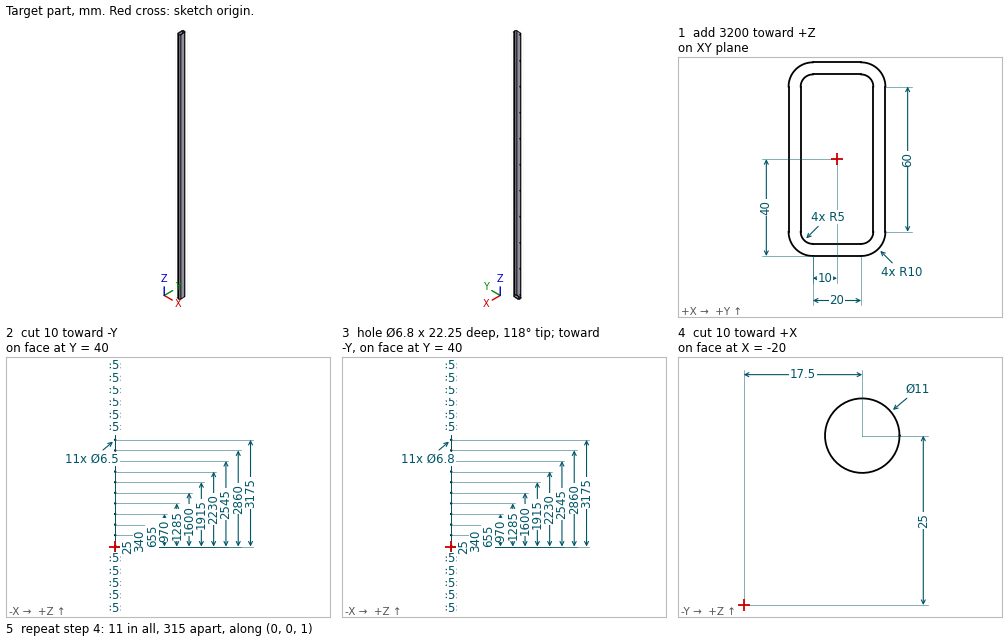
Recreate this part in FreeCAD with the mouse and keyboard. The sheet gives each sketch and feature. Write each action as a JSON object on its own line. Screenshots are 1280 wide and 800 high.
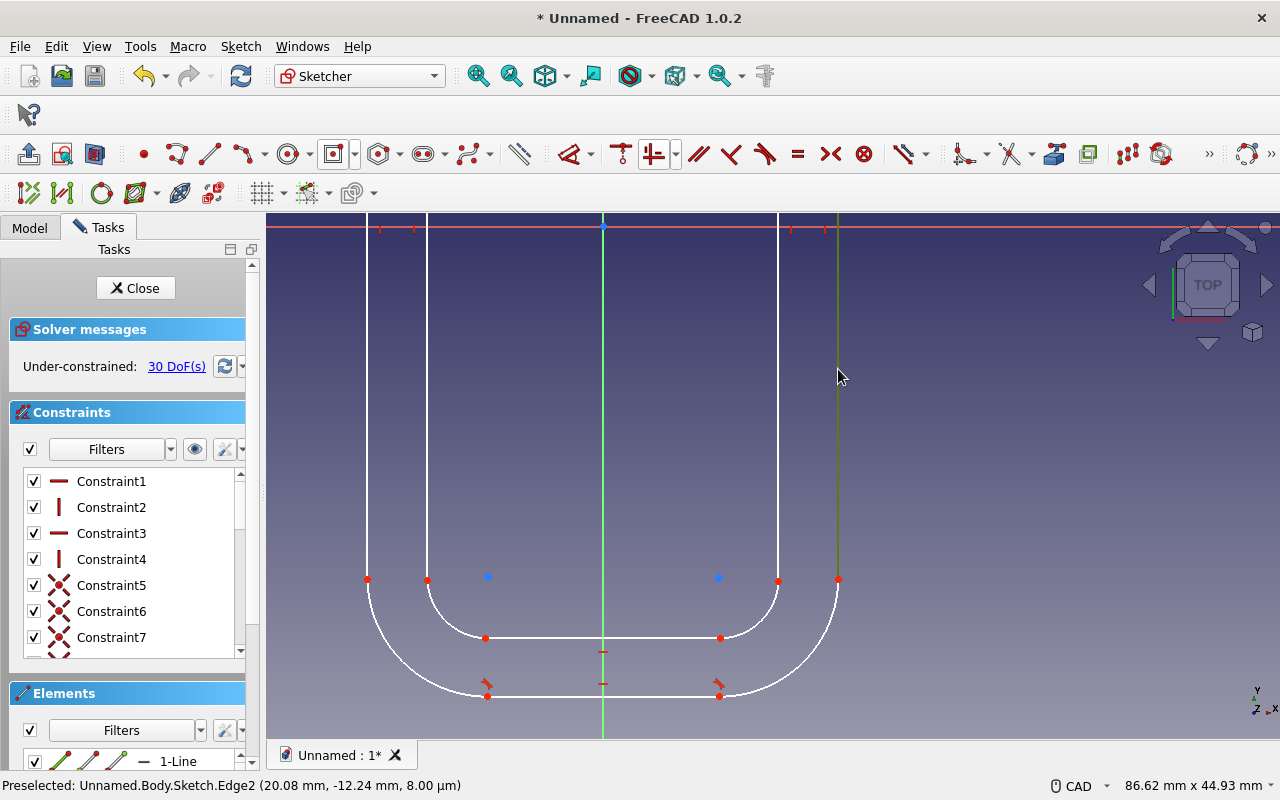
{"action": "left_click", "coordinate": [773, 684]}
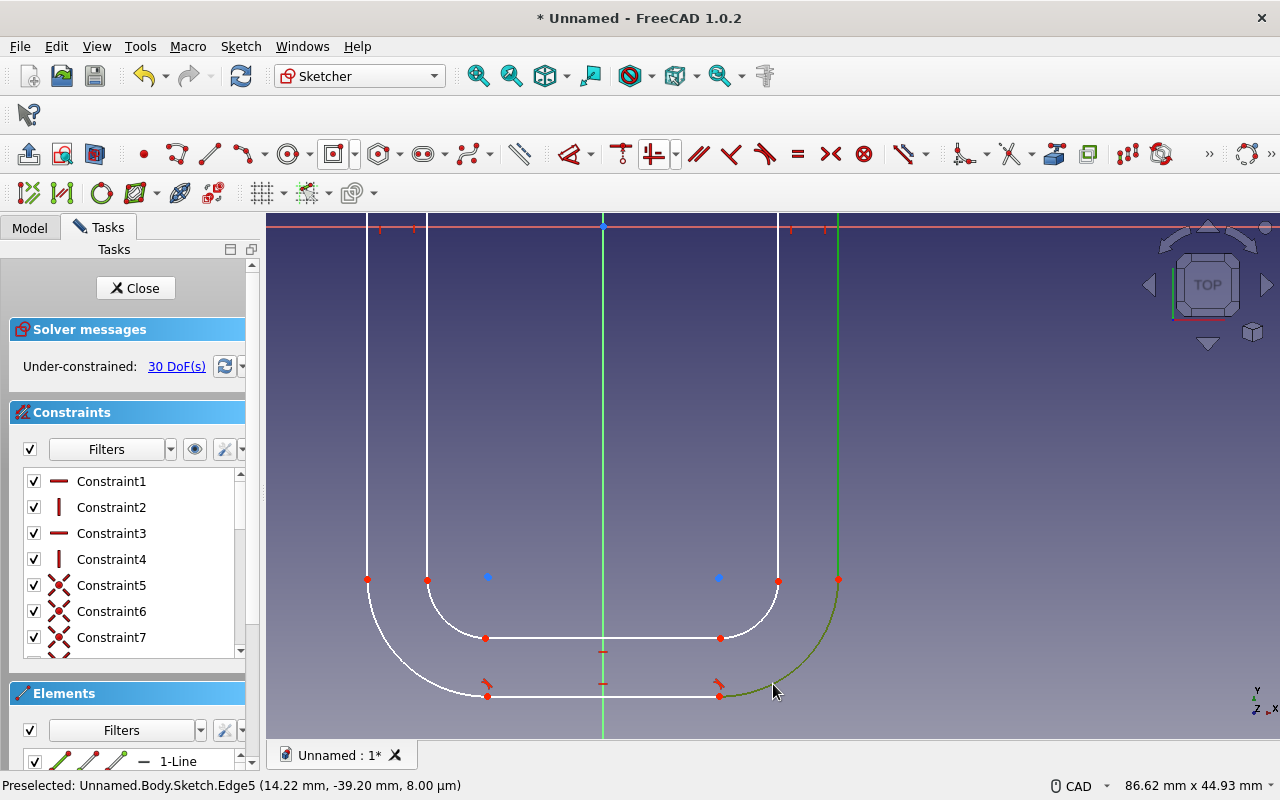
{"action": "left_click", "coordinate": [765, 154]}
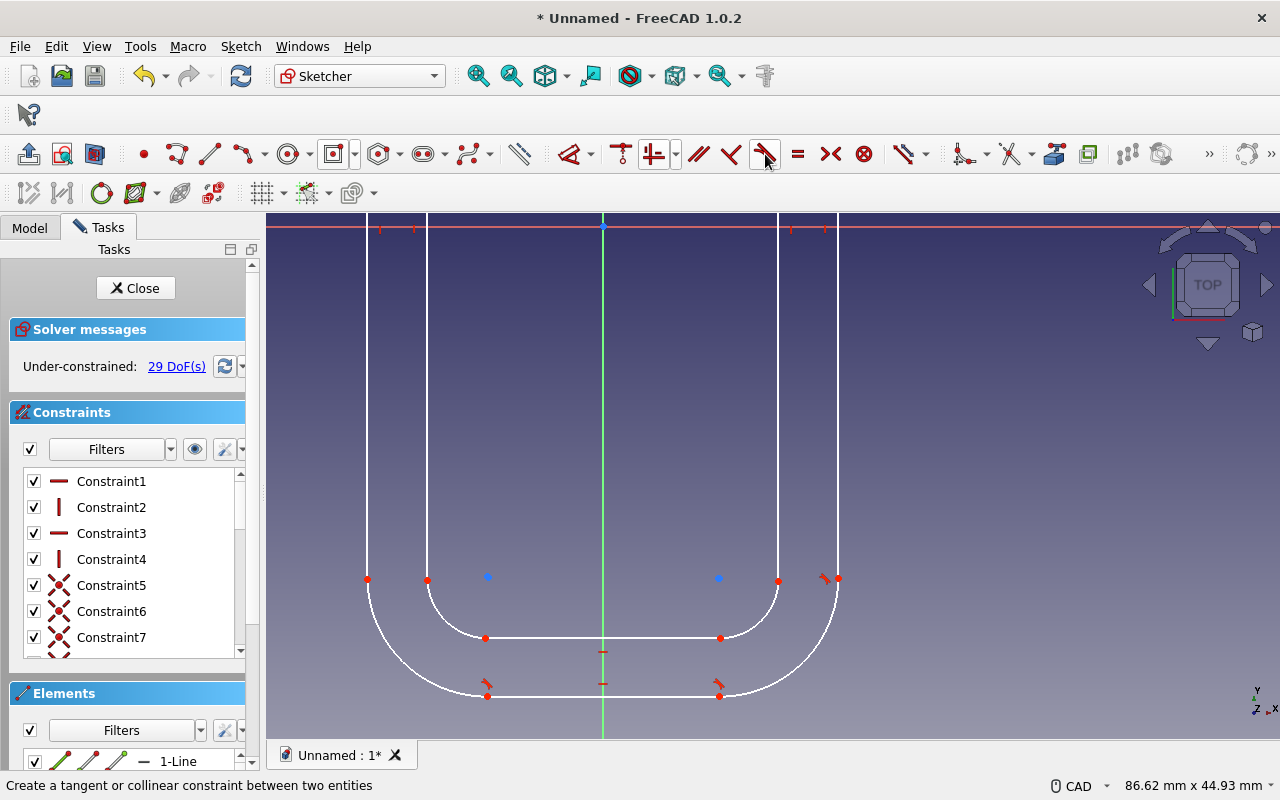
{"action": "left_click", "coordinate": [838, 368]}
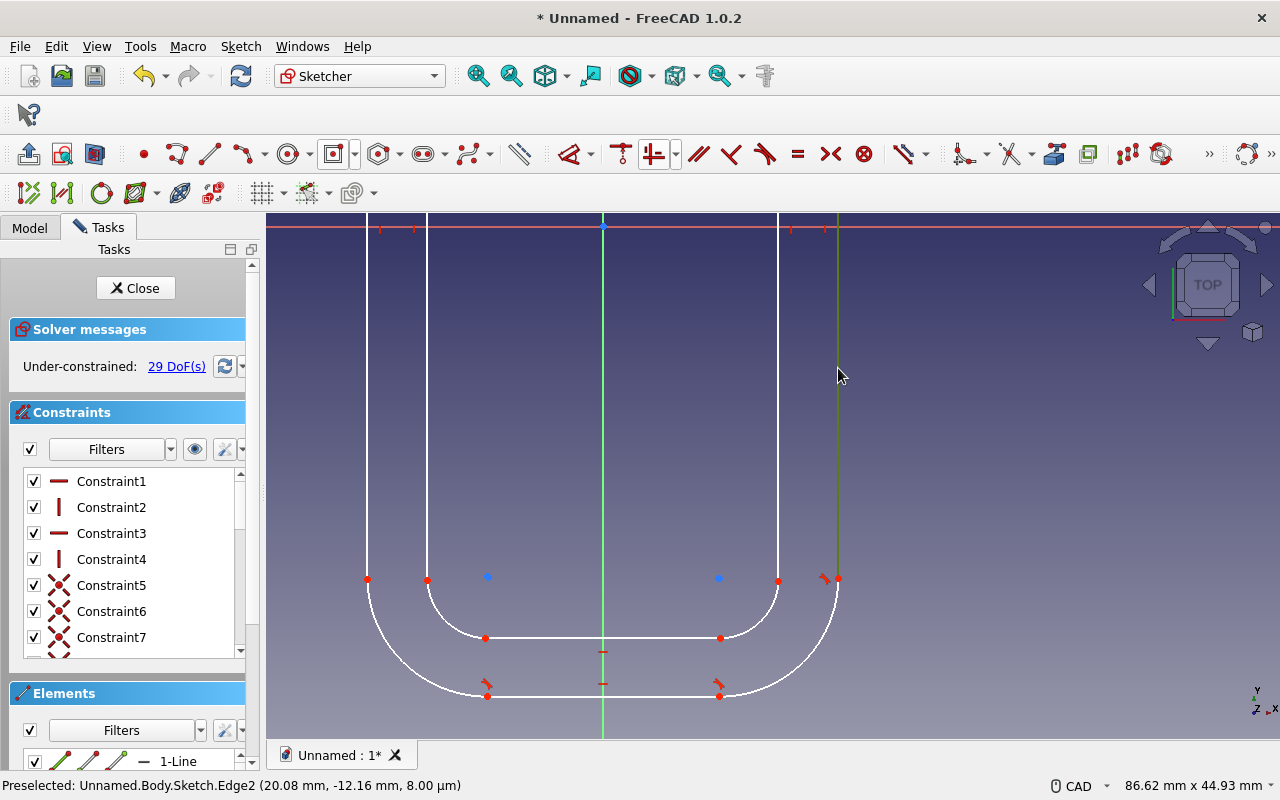
{"action": "scroll", "coordinate": [763, 621], "scroll_direction": "down", "scroll_amount": 5}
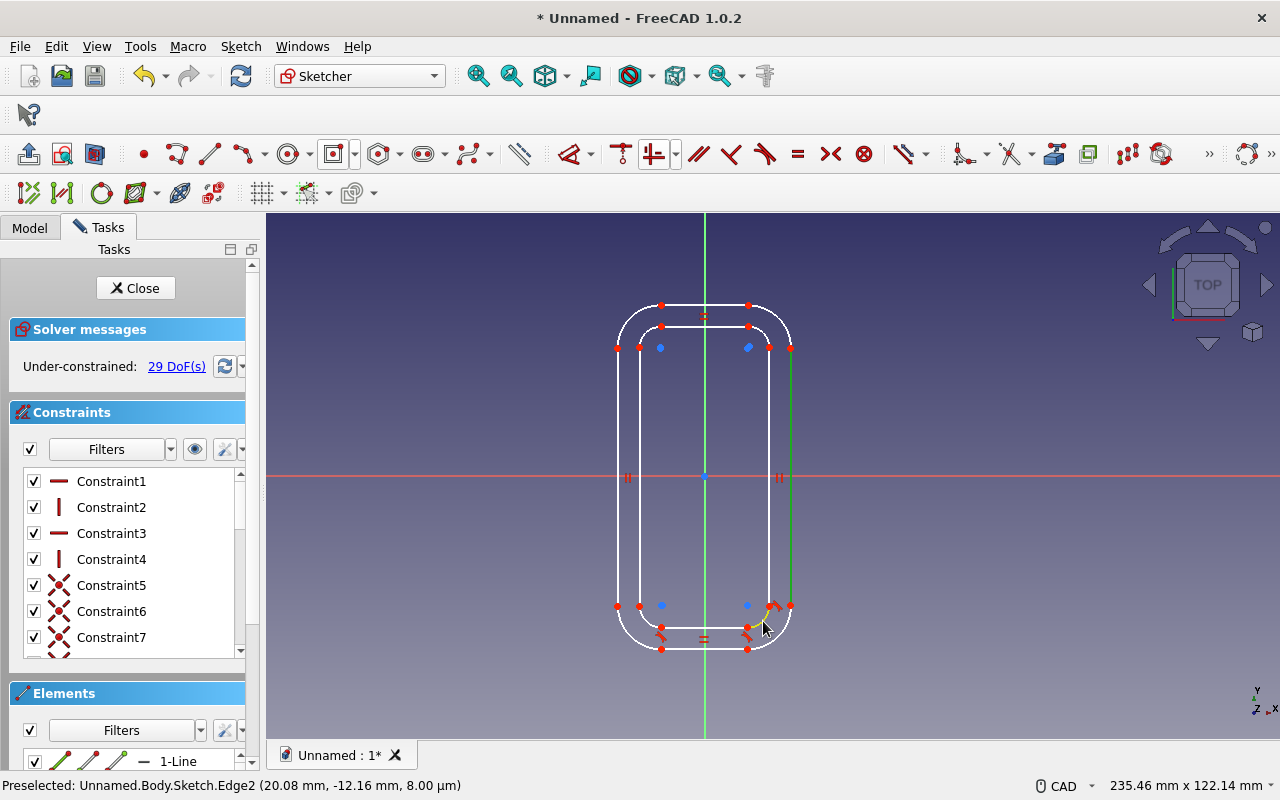
{"action": "left_click", "coordinate": [786, 329]}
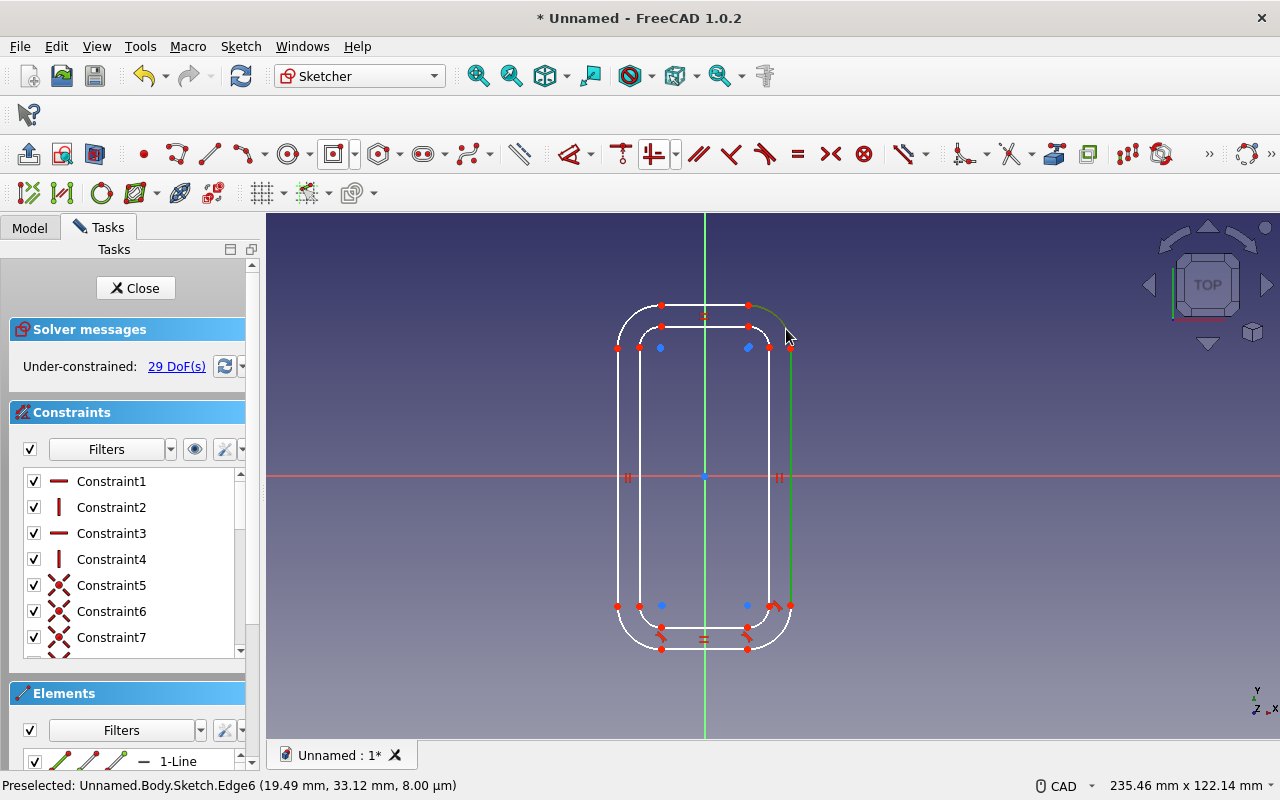
{"action": "left_click", "coordinate": [765, 154]}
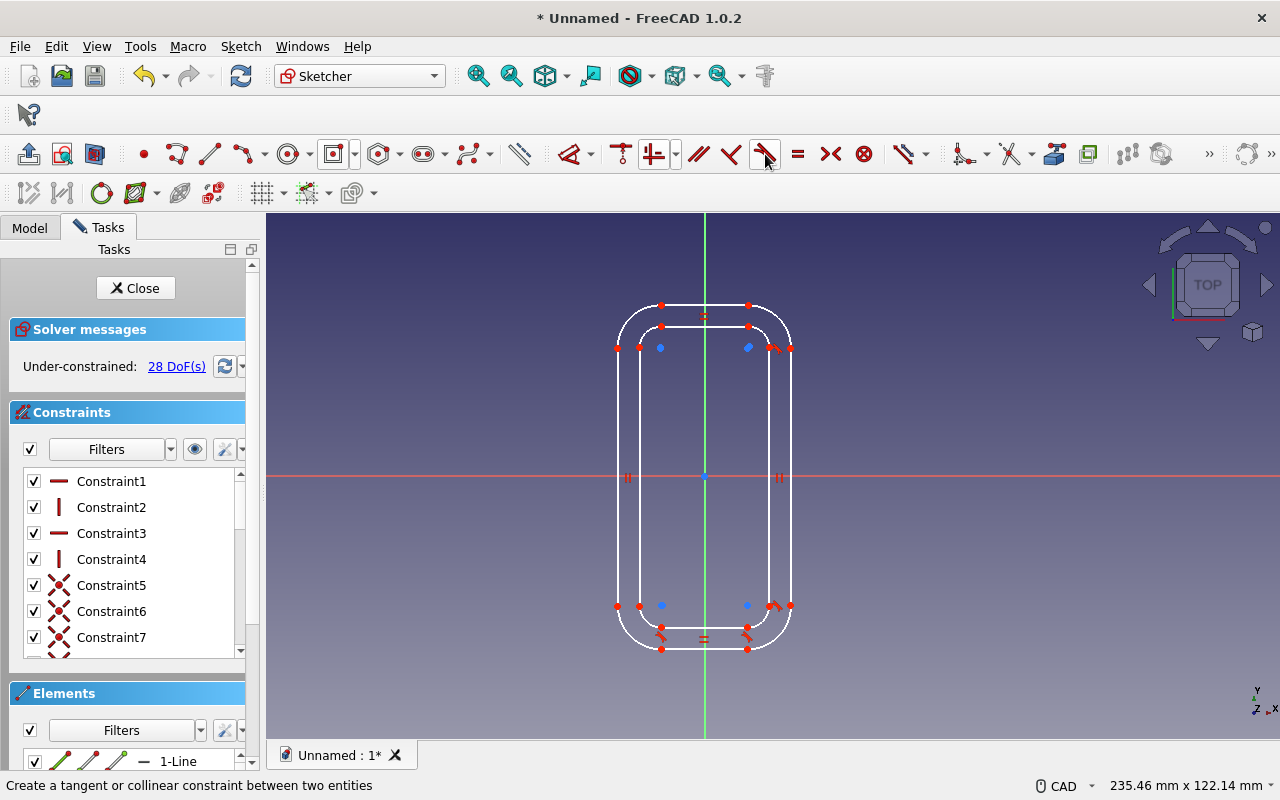
{"action": "left_click", "coordinate": [722, 305]}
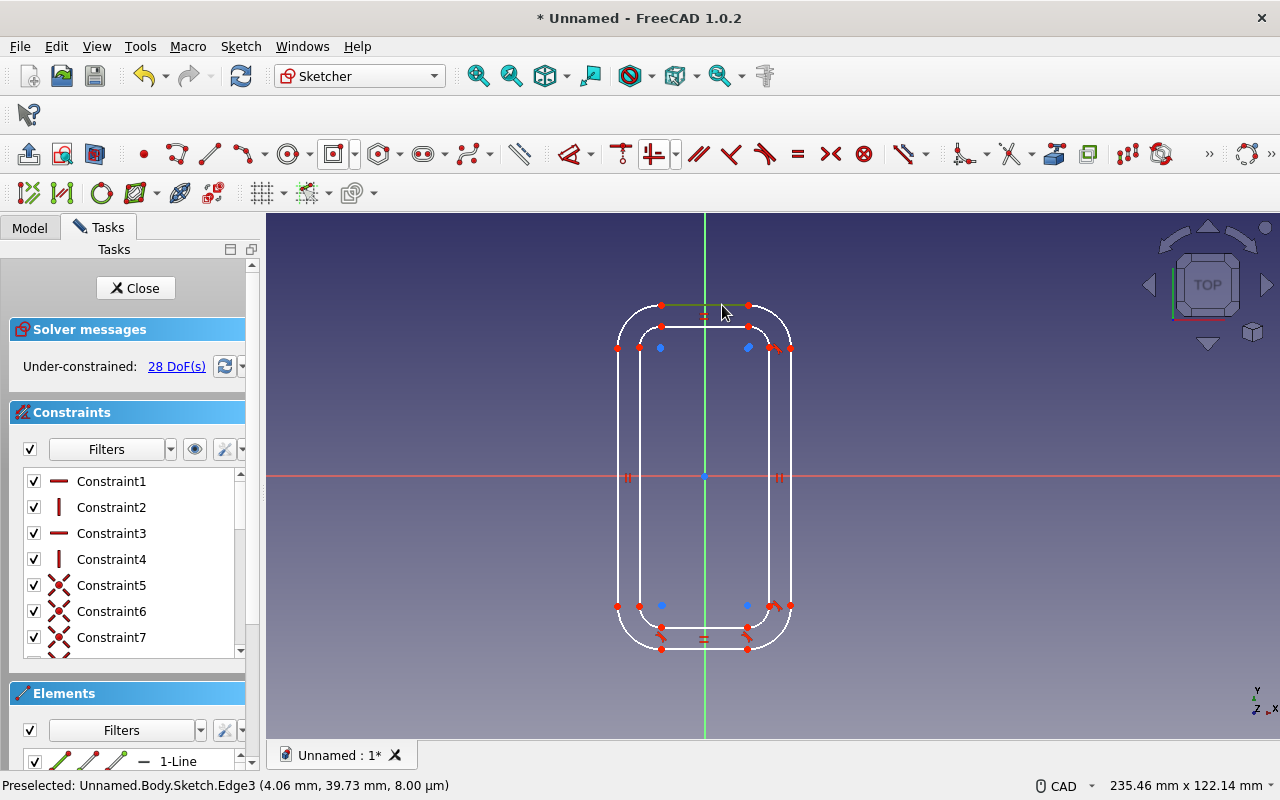
{"action": "left_click", "coordinate": [786, 329]}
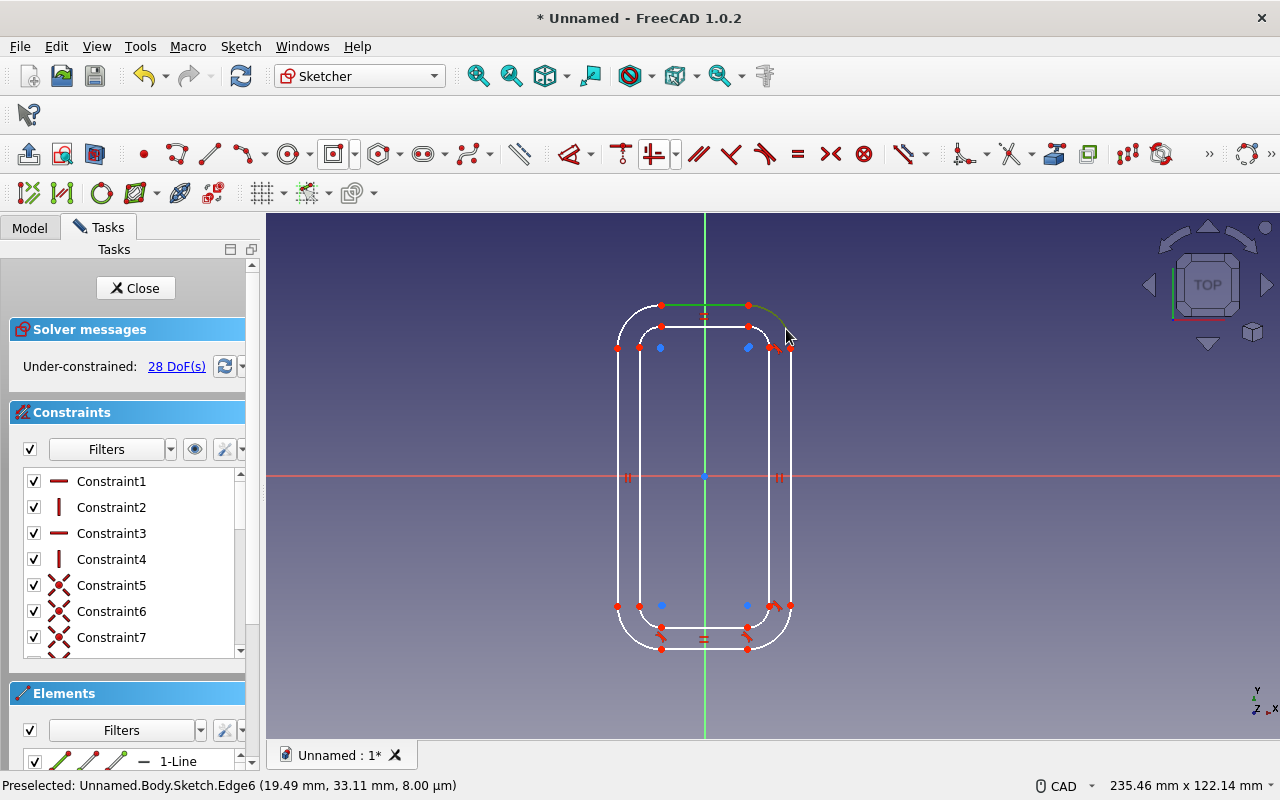
{"action": "left_click", "coordinate": [765, 154]}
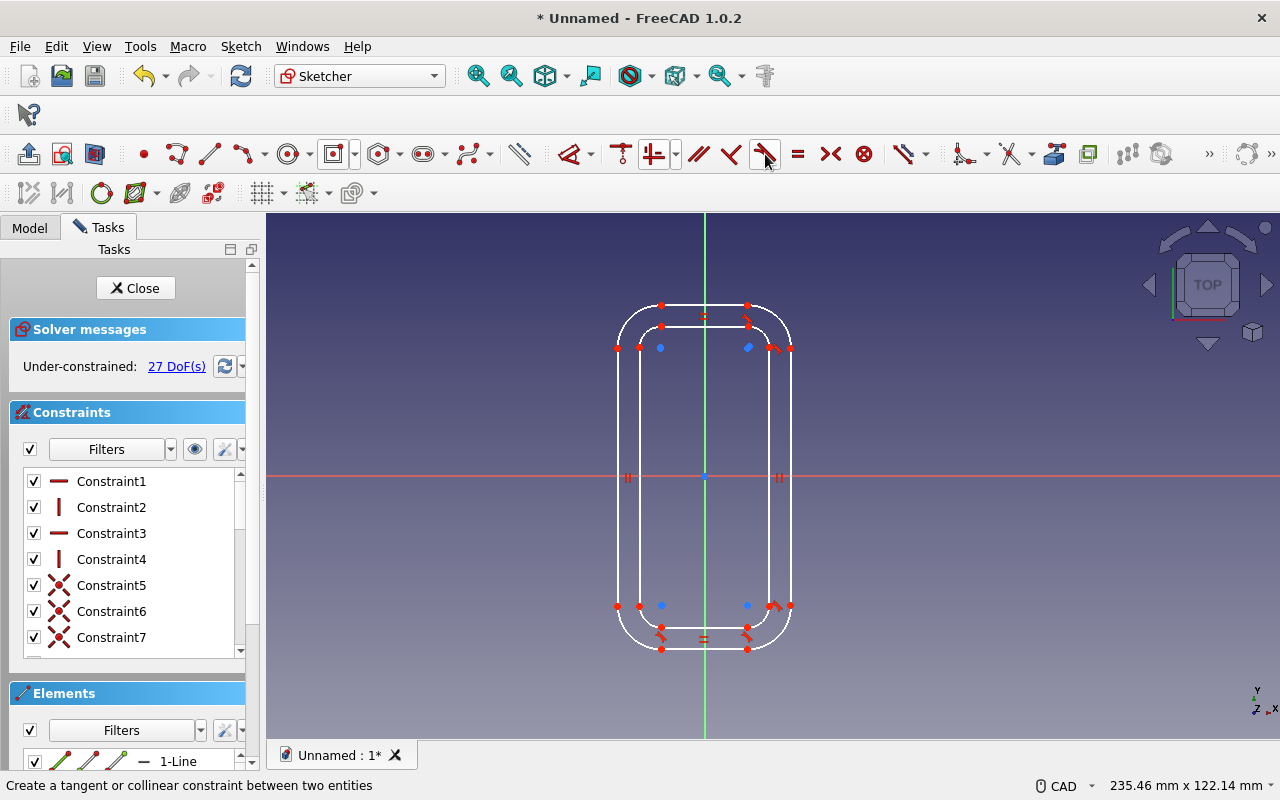
{"action": "left_click", "coordinate": [722, 305]}